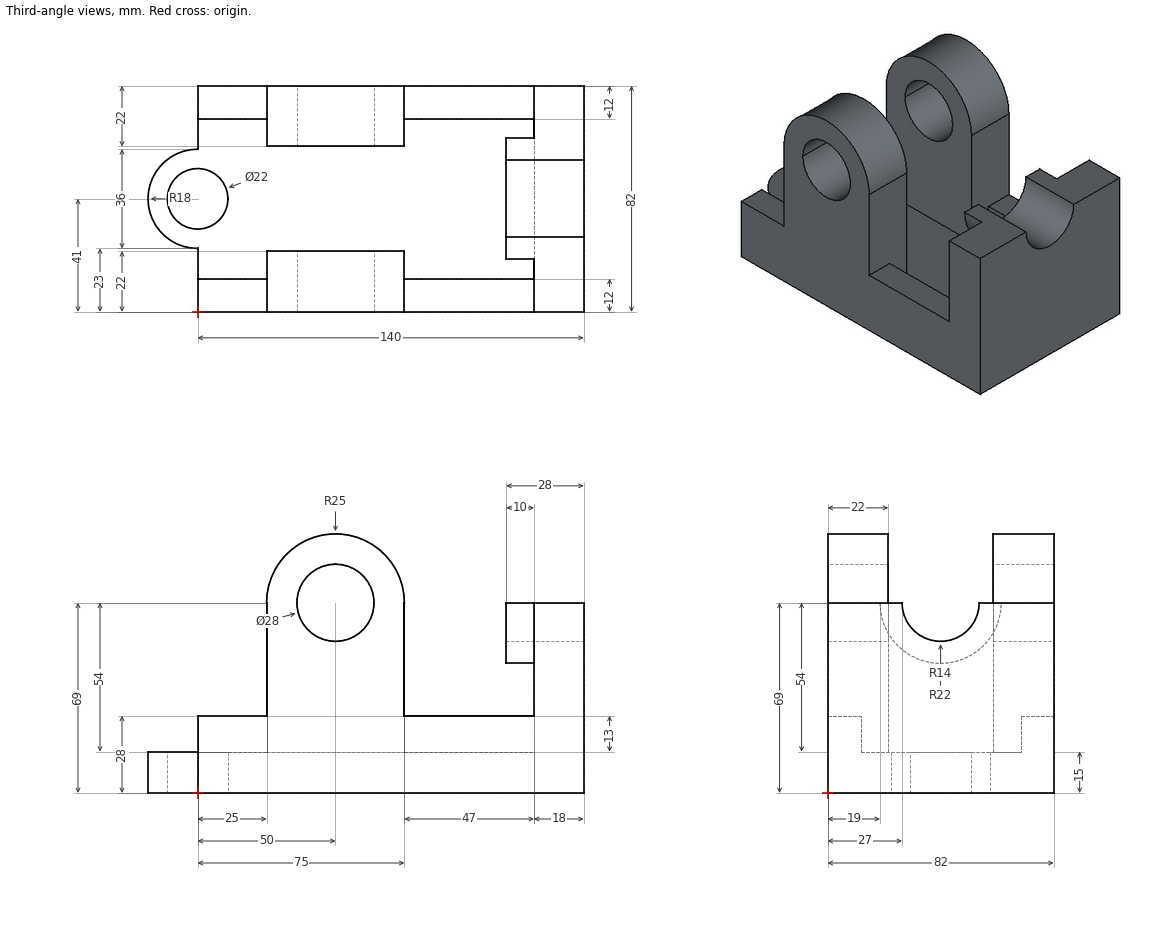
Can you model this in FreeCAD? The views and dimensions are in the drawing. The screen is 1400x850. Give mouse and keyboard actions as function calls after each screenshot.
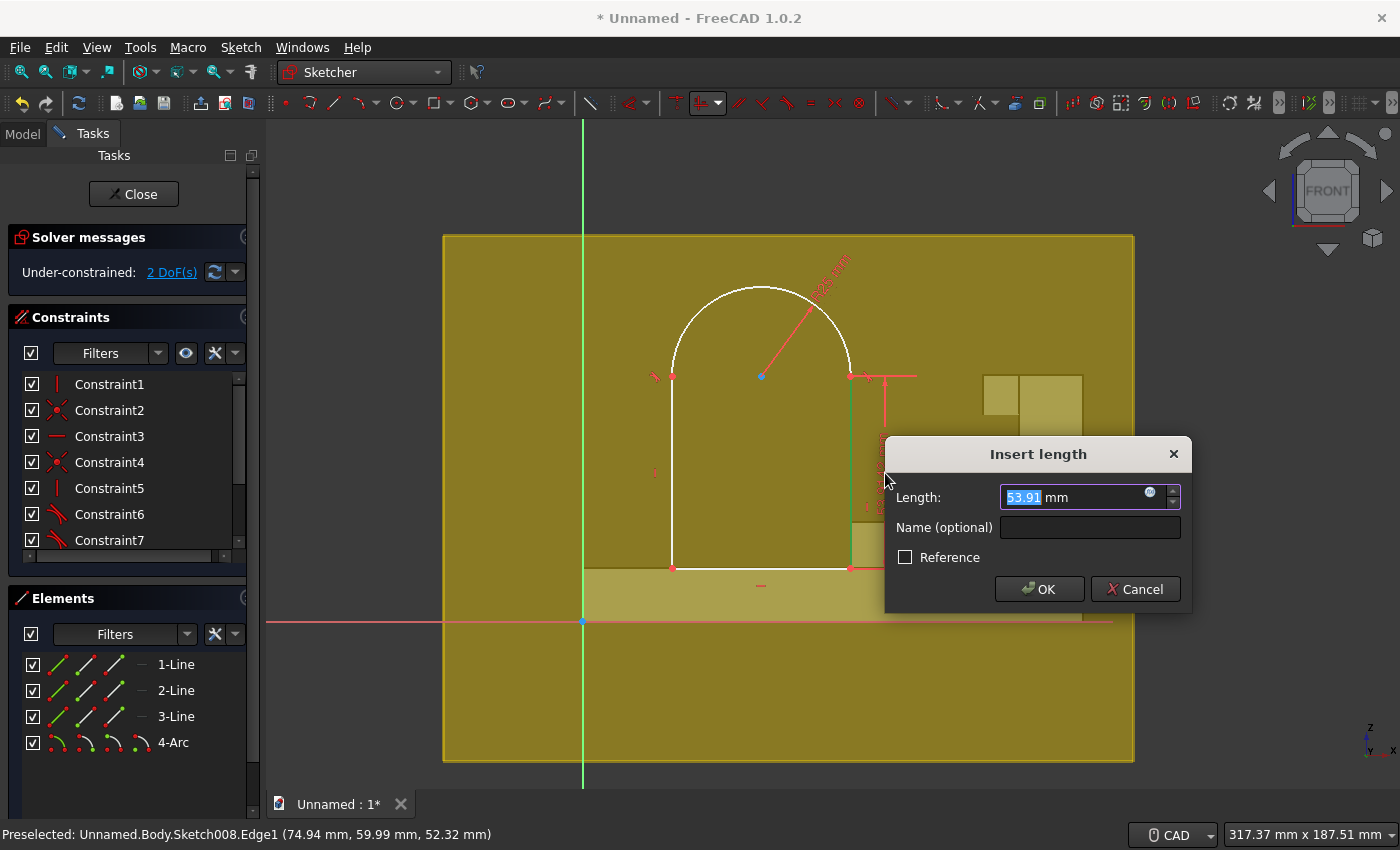
text(54)
key(Return)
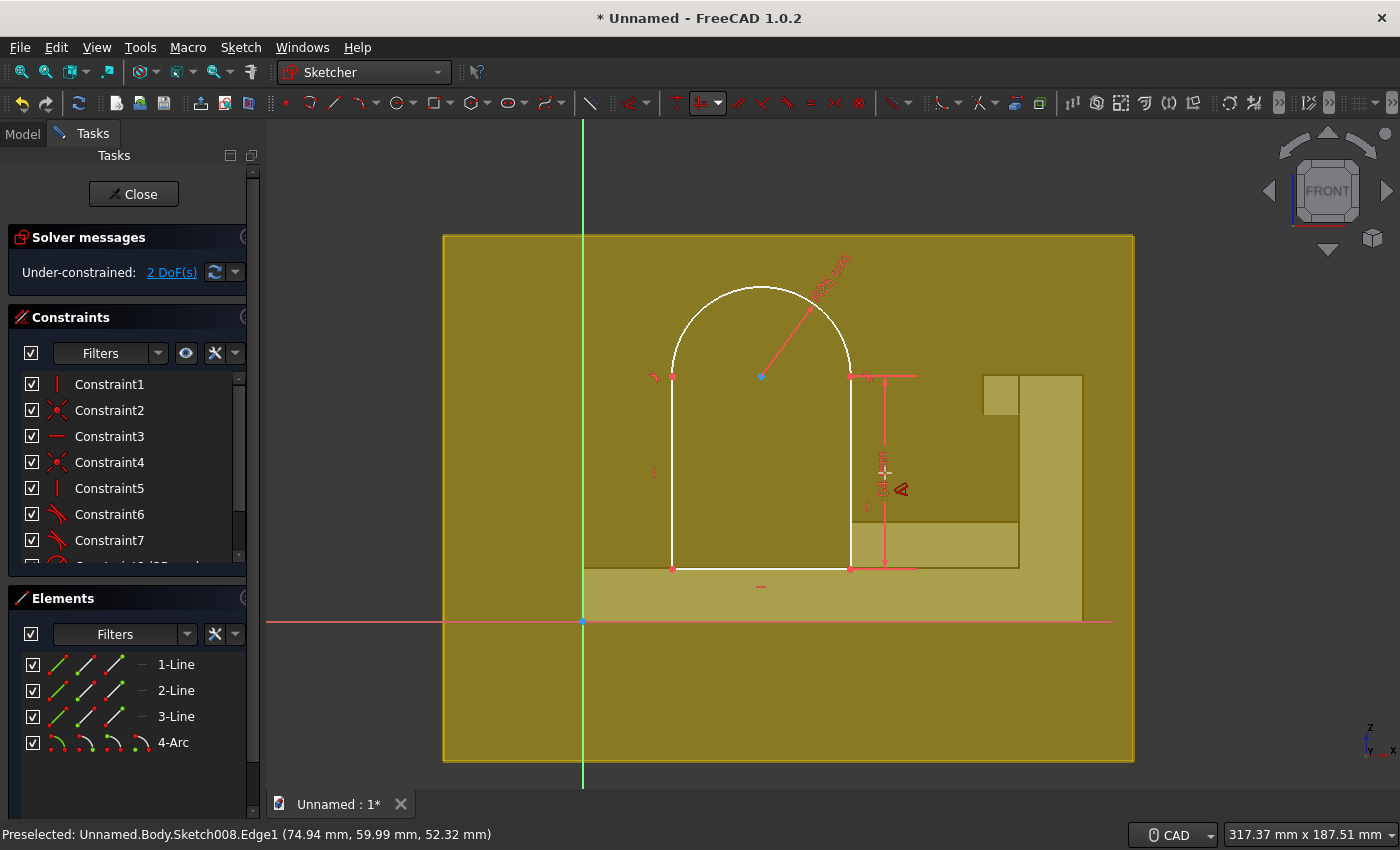
click(851, 376)
click(717, 656)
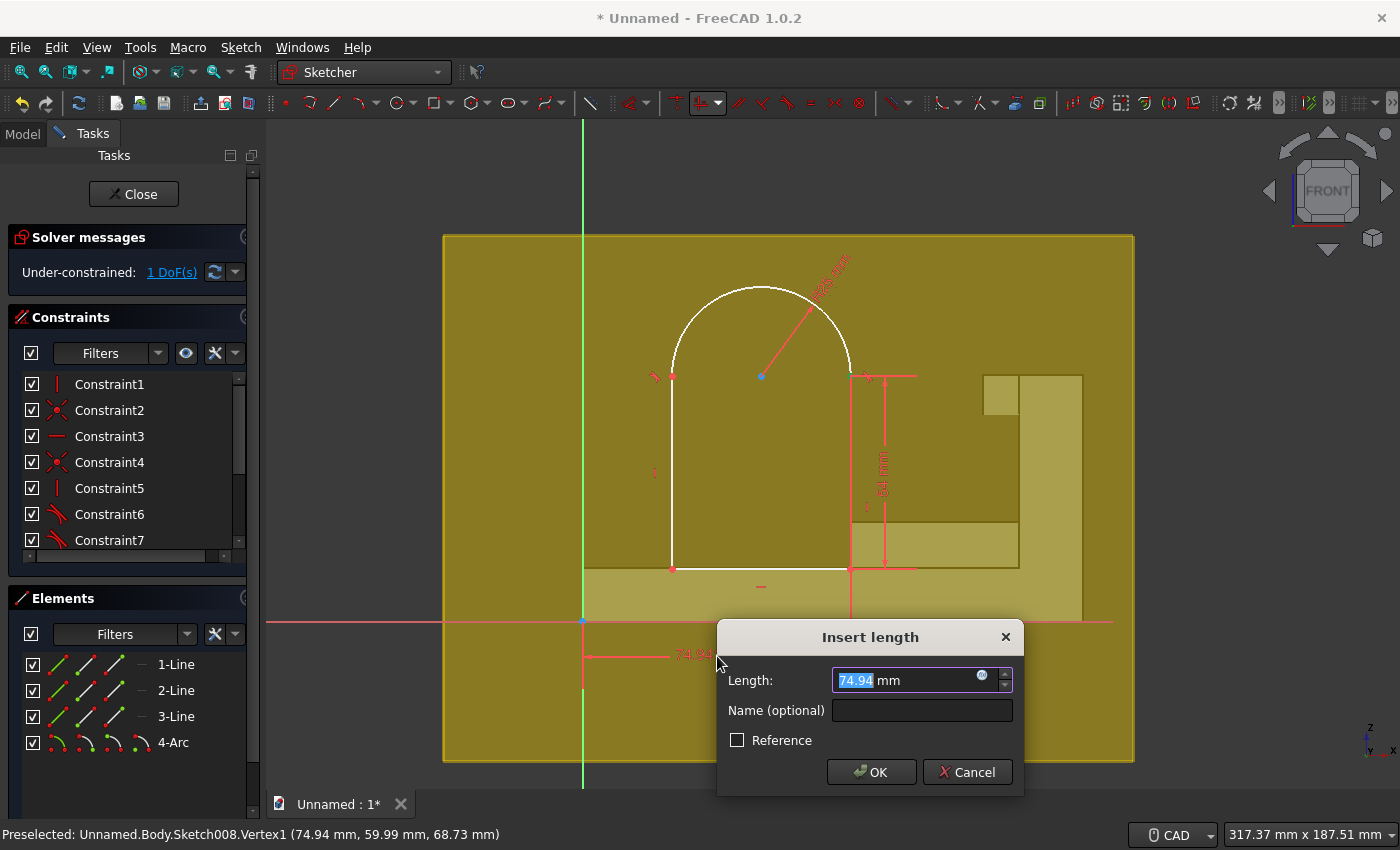
text(75)
key(Return)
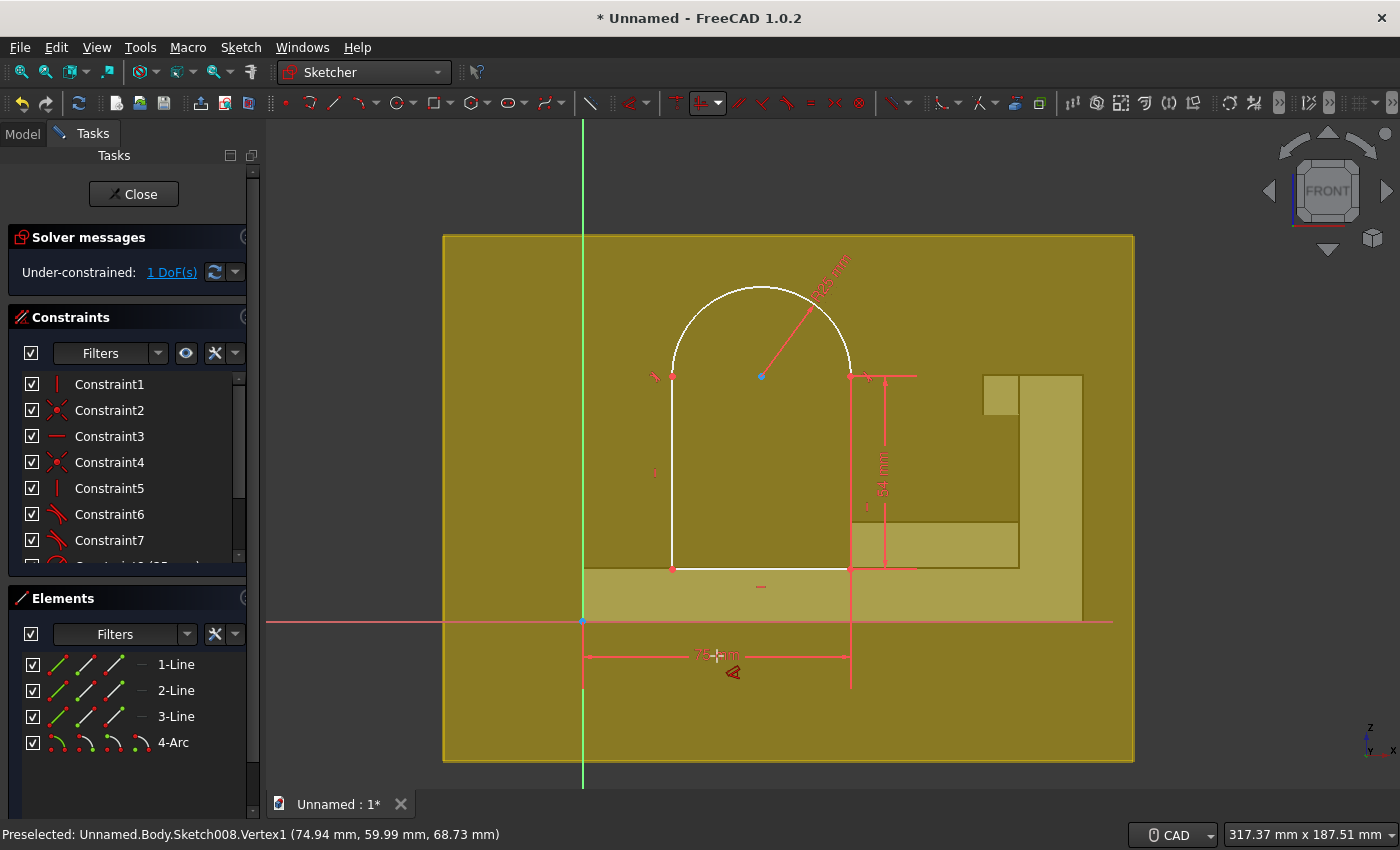
click(851, 376)
click(885, 499)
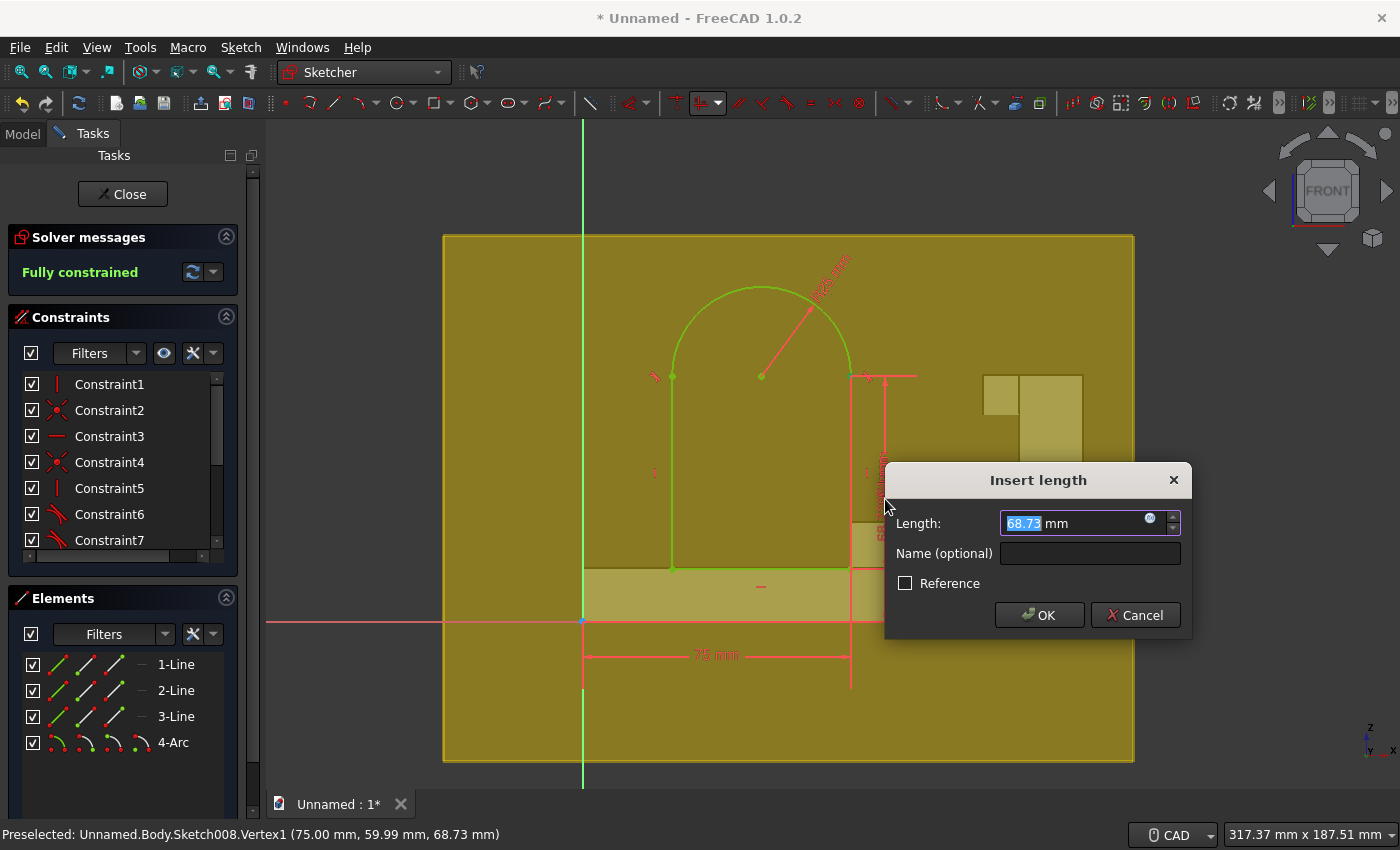
text(69)
key(Return)
key(Escape)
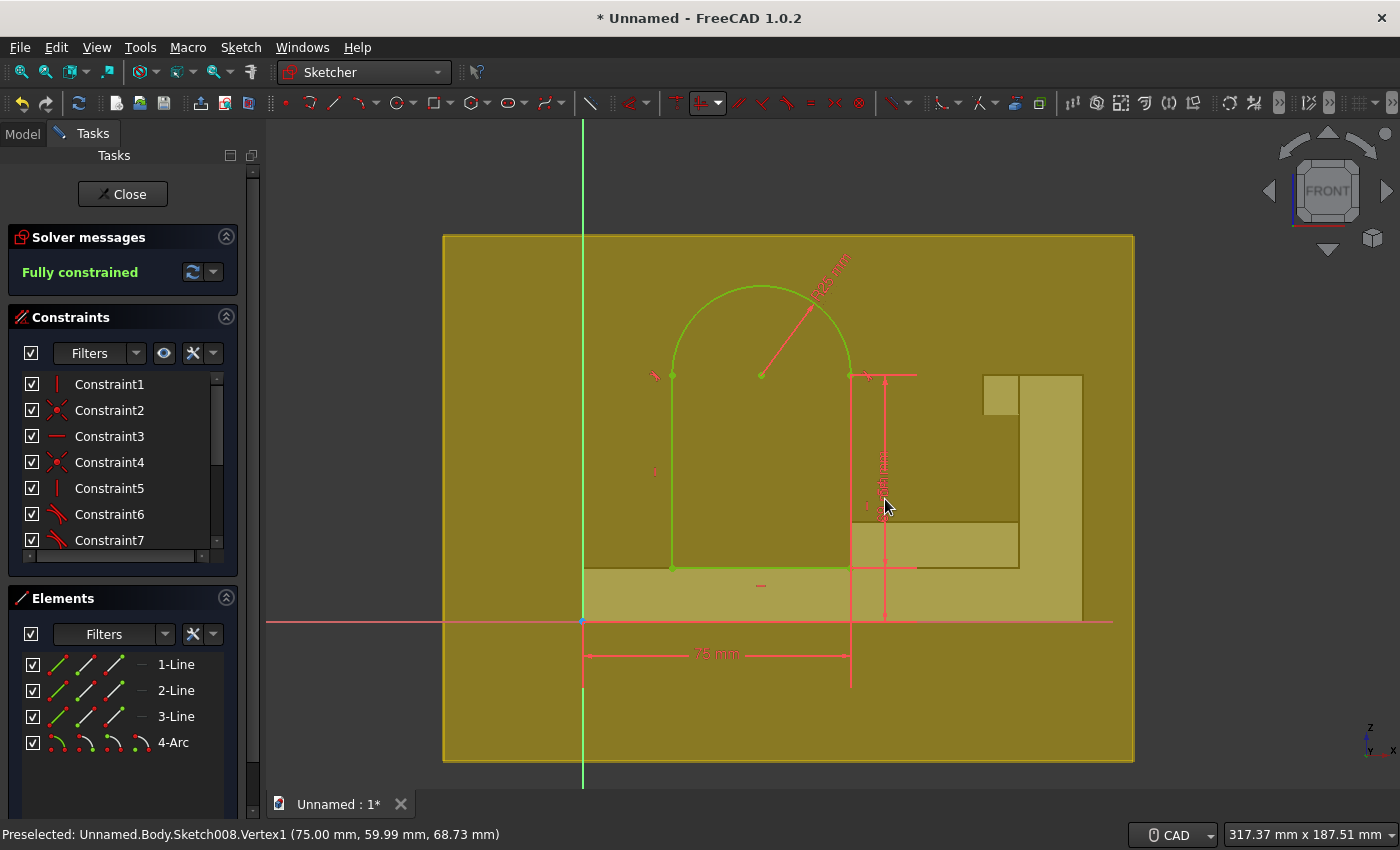
click(123, 194)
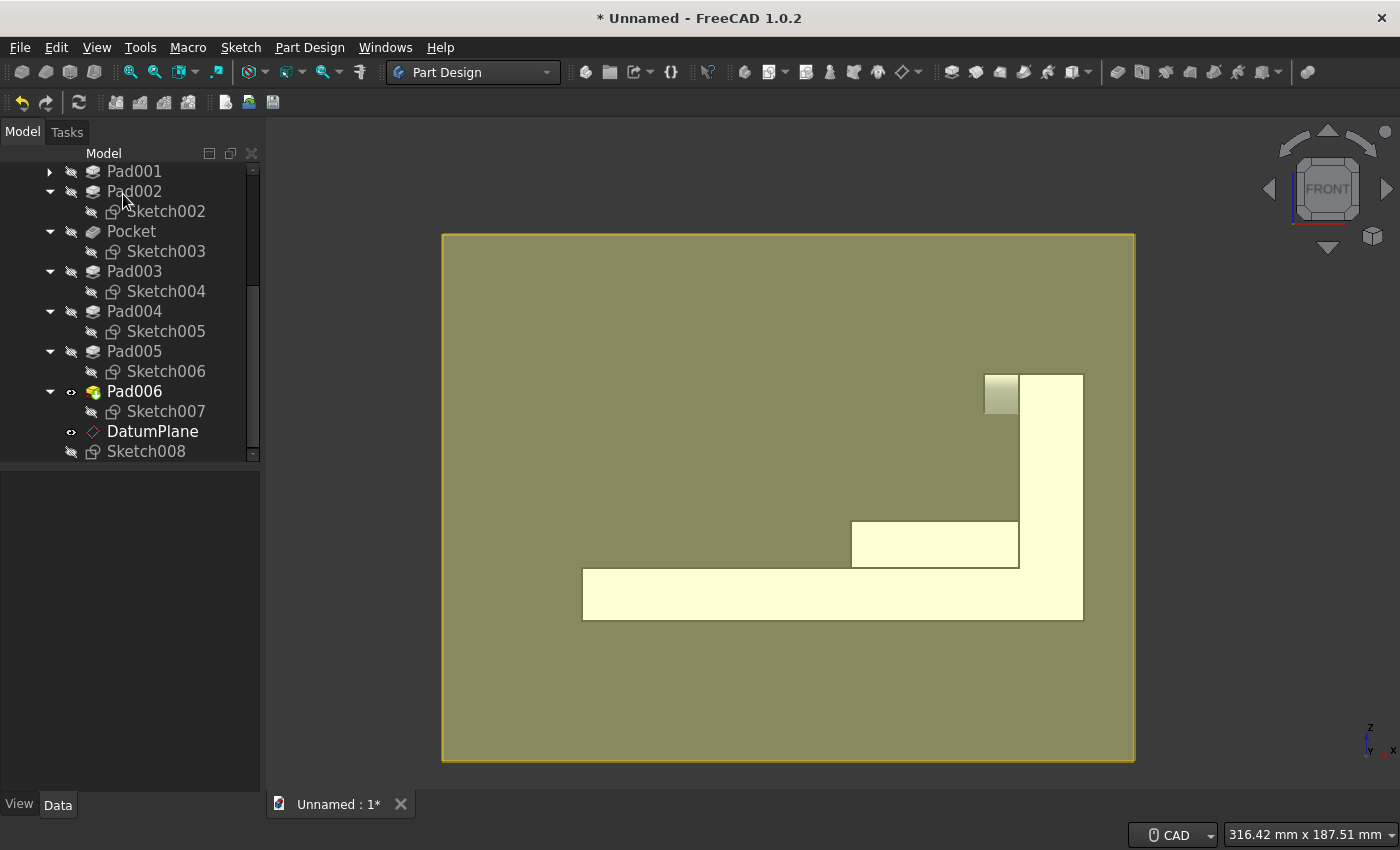
click(952, 72)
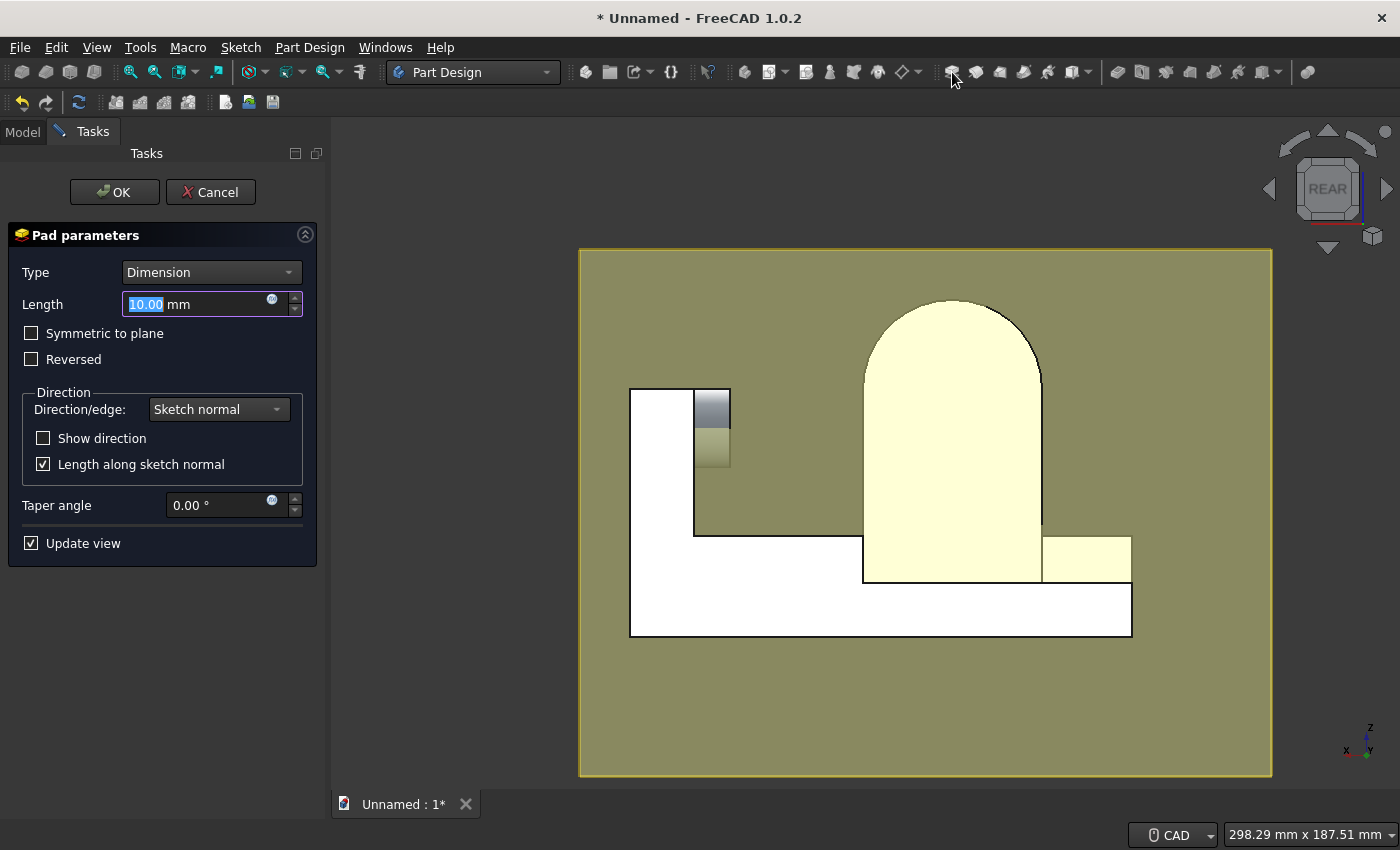
text(22)
key(Tab)